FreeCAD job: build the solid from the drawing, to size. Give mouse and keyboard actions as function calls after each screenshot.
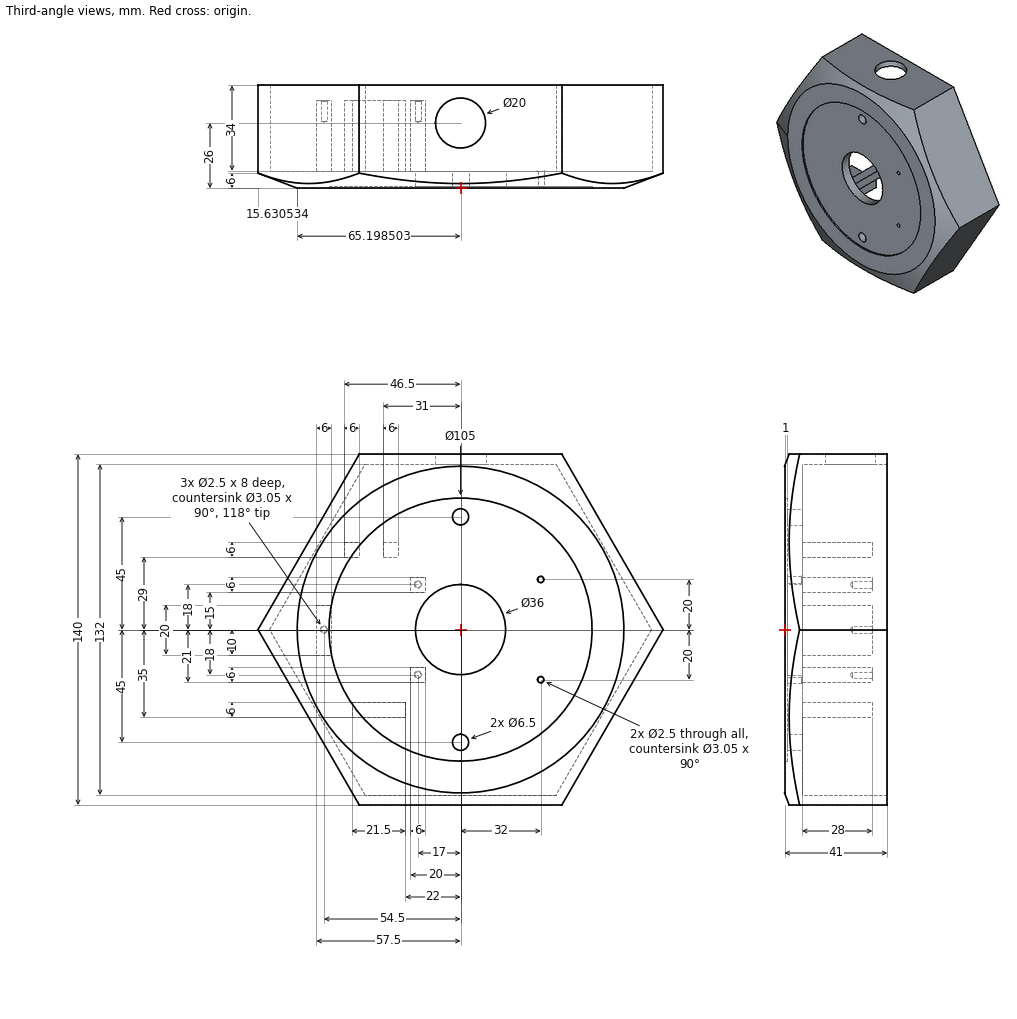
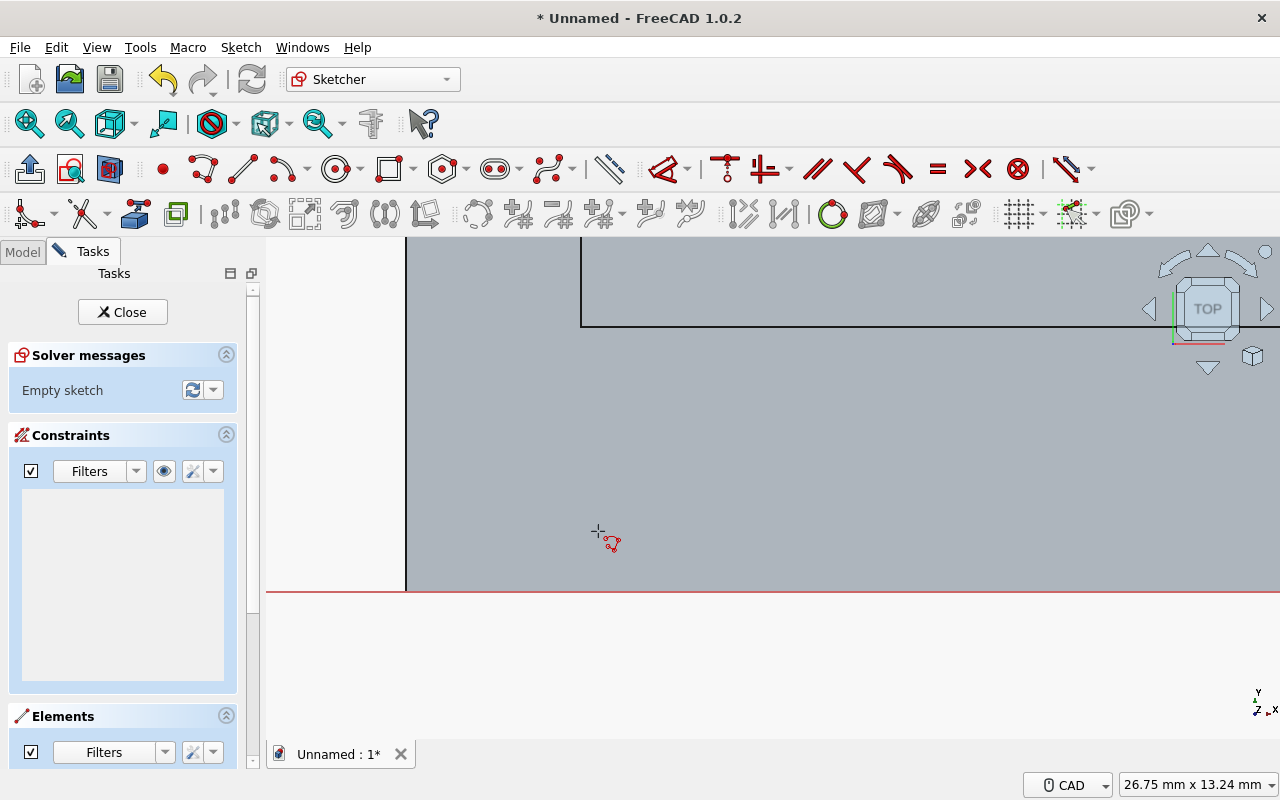
click(999, 592)
click(406, 365)
click(406, 583)
click(999, 592)
key(Escape)
key(Escape)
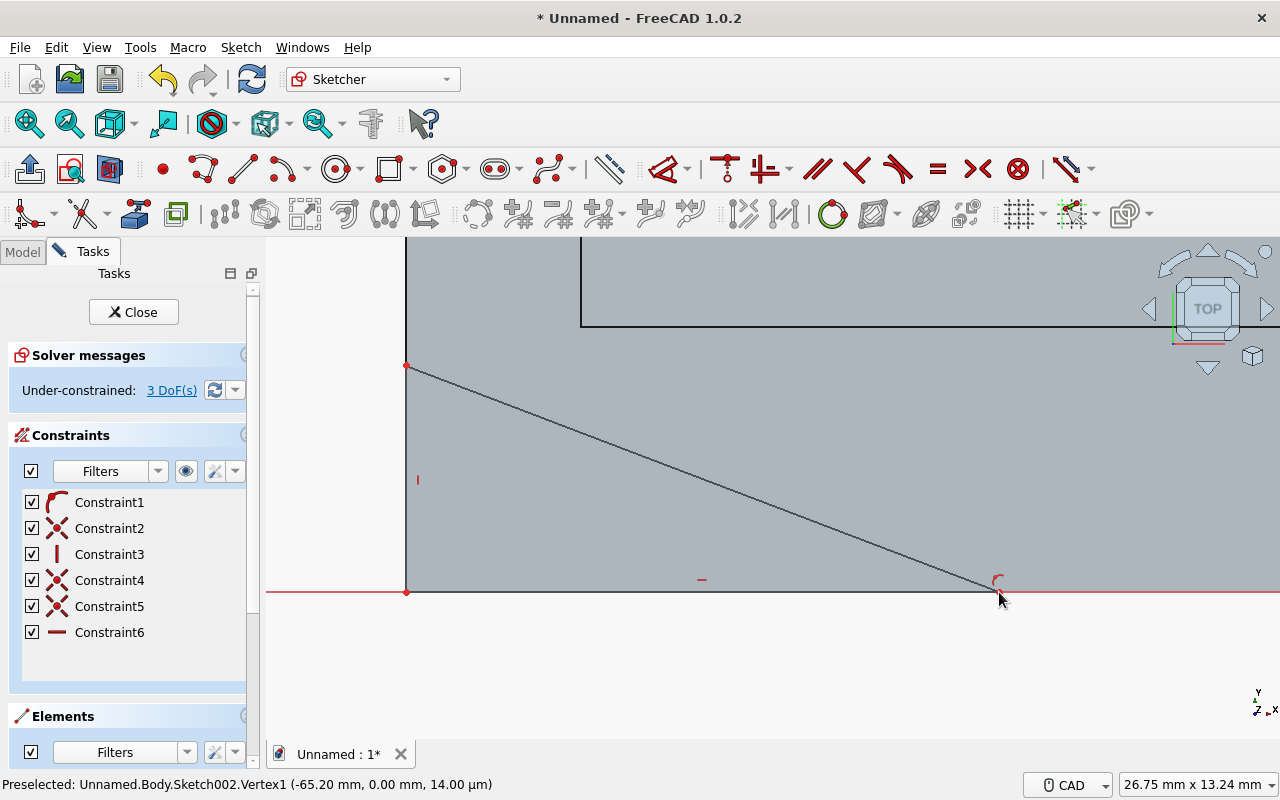
click(406, 434)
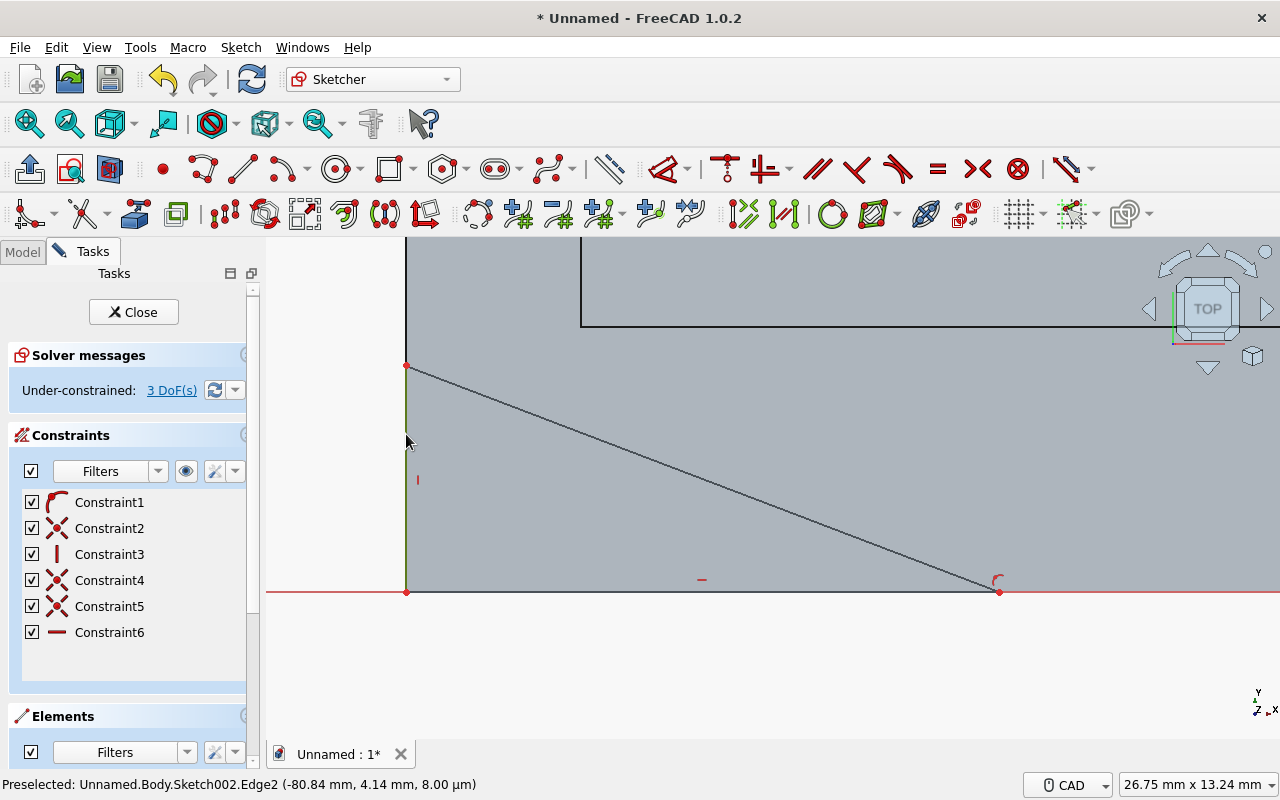
key(i)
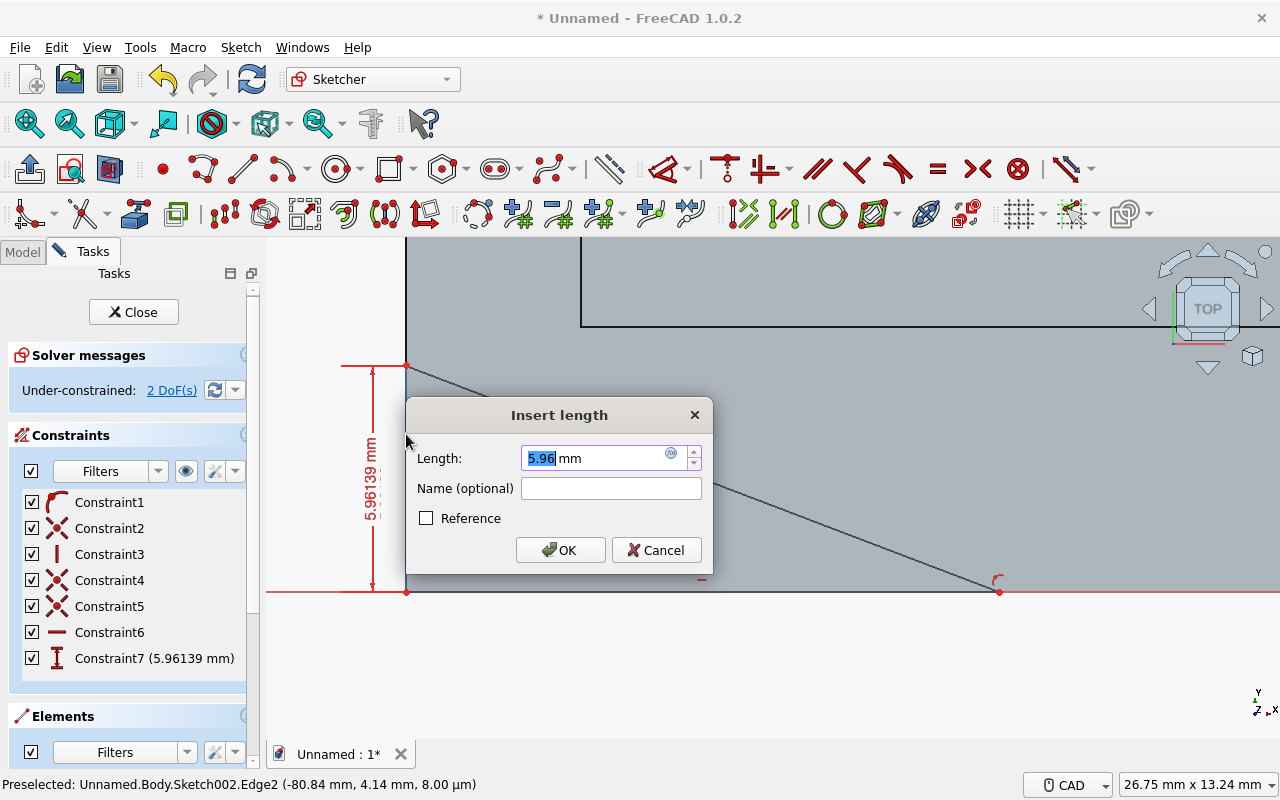
text(6)
key(Return)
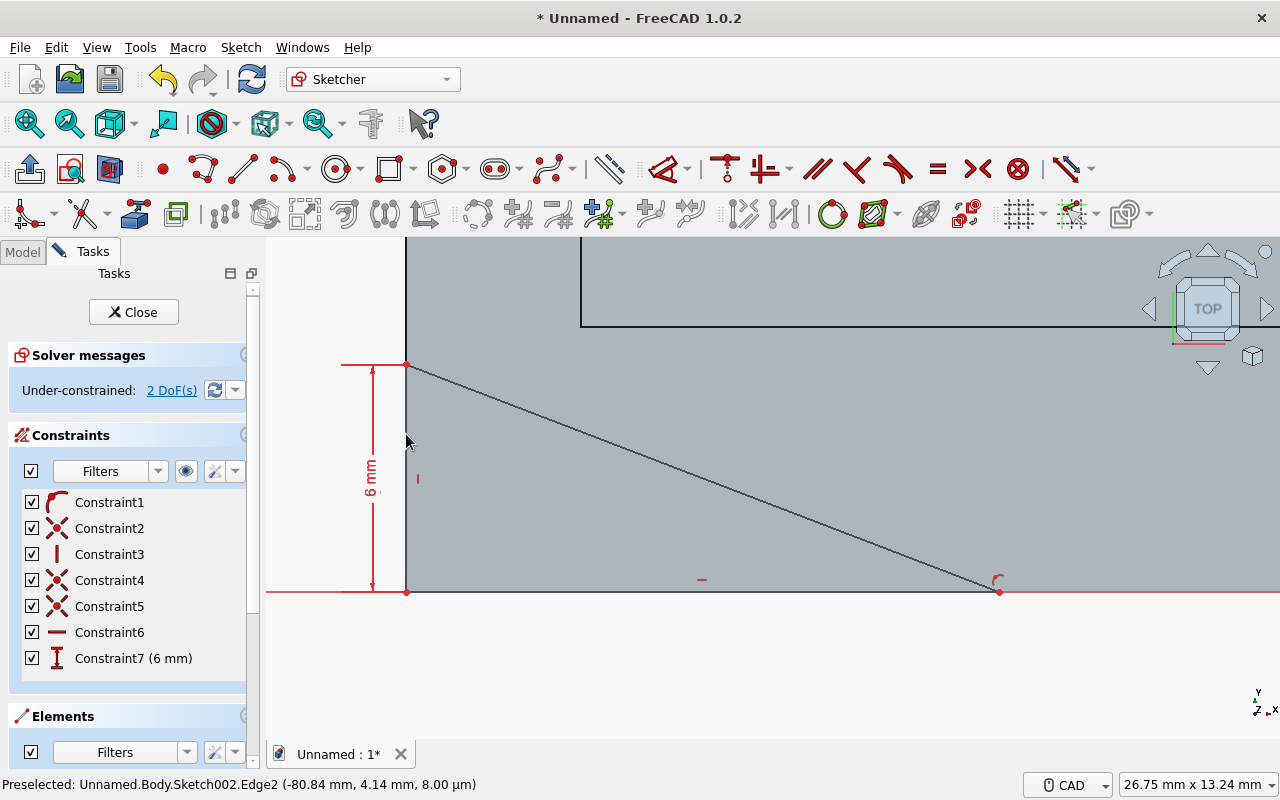
click(584, 592)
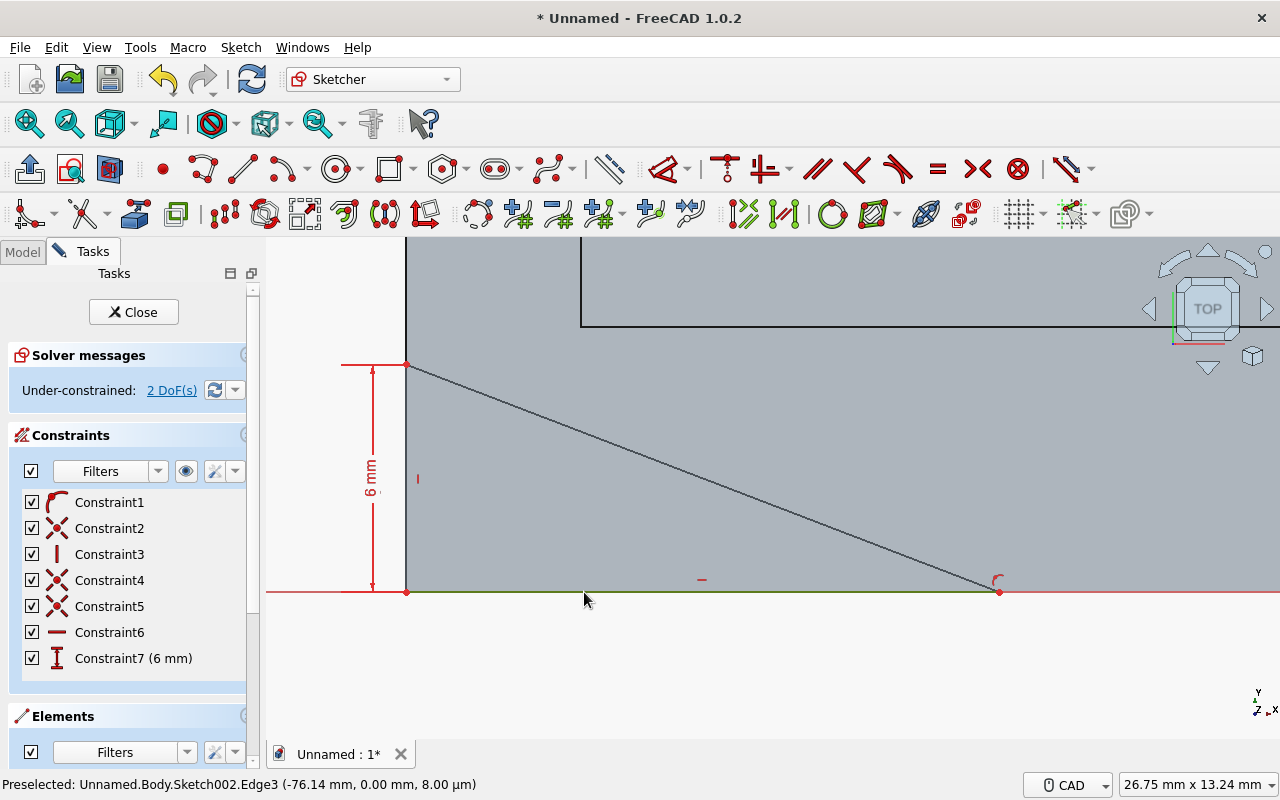
key(l)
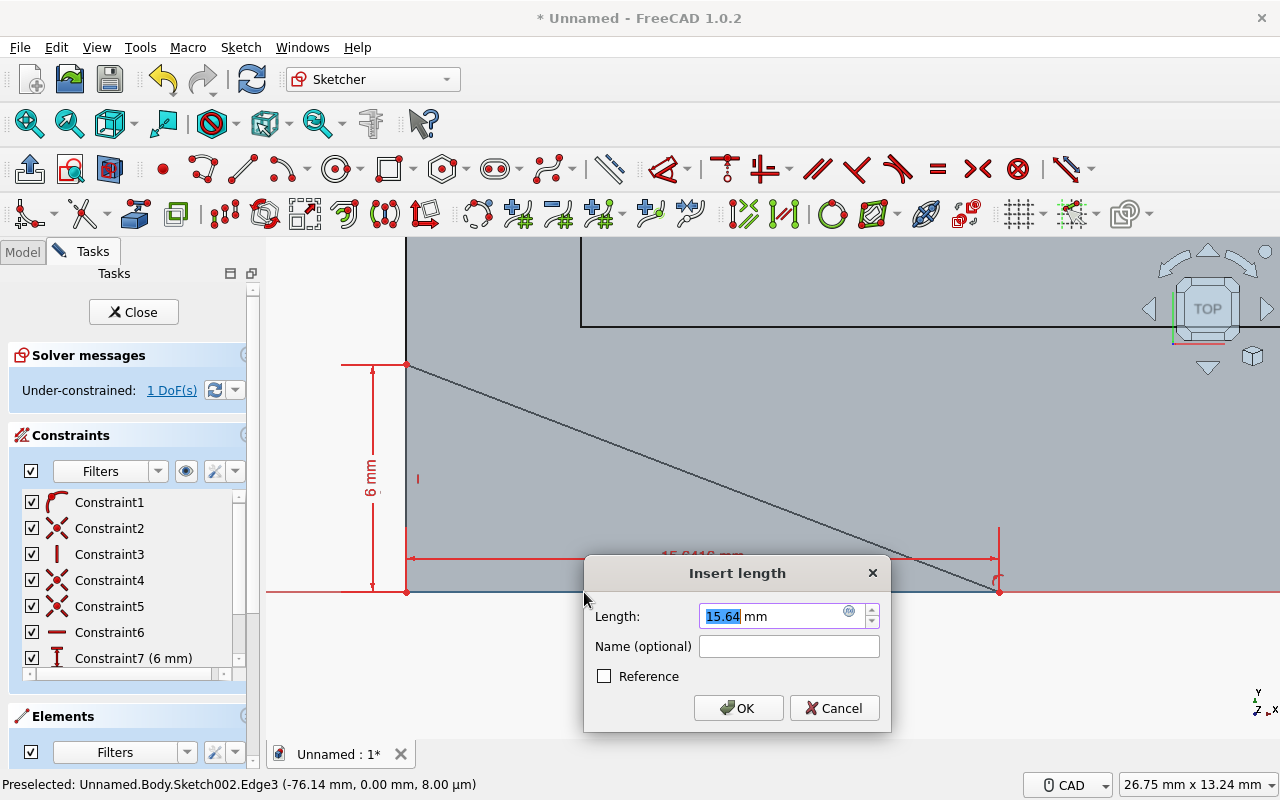
text(15.630534)
key(Return)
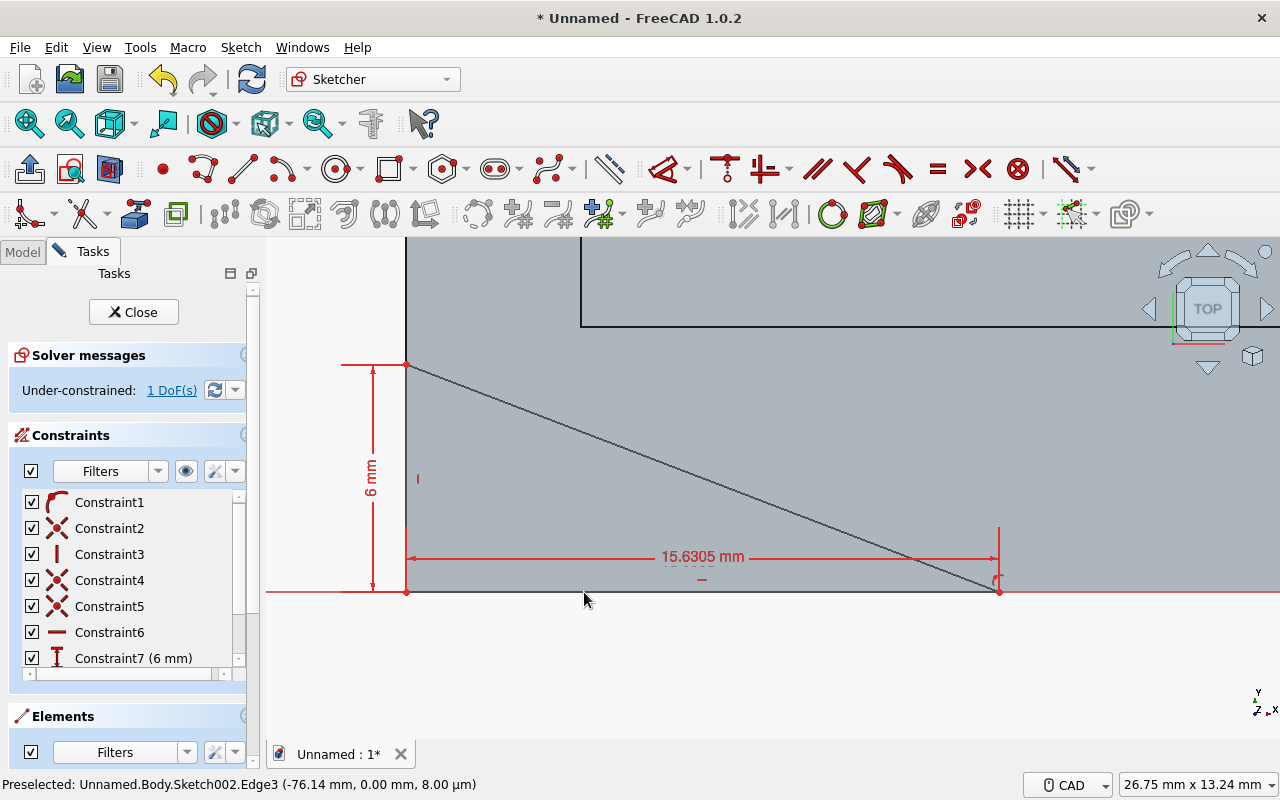
click(999, 592)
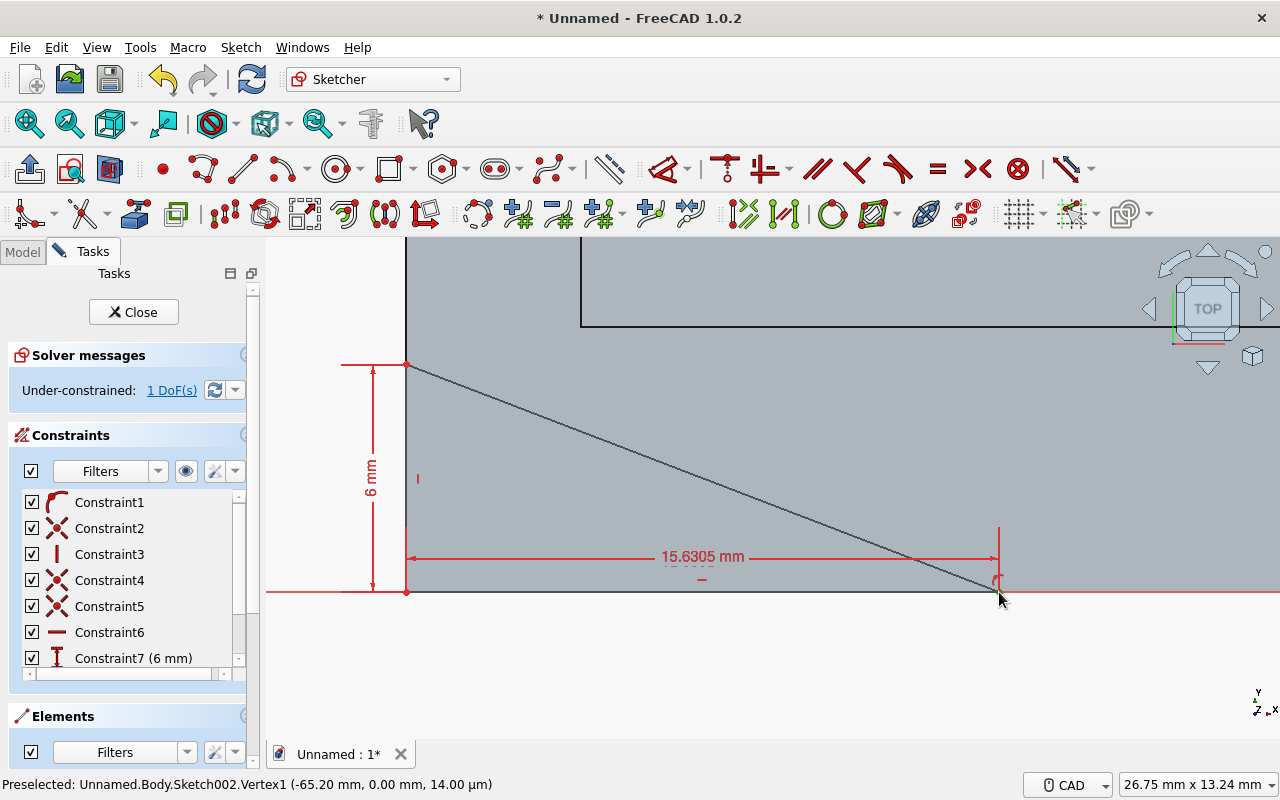
key(l)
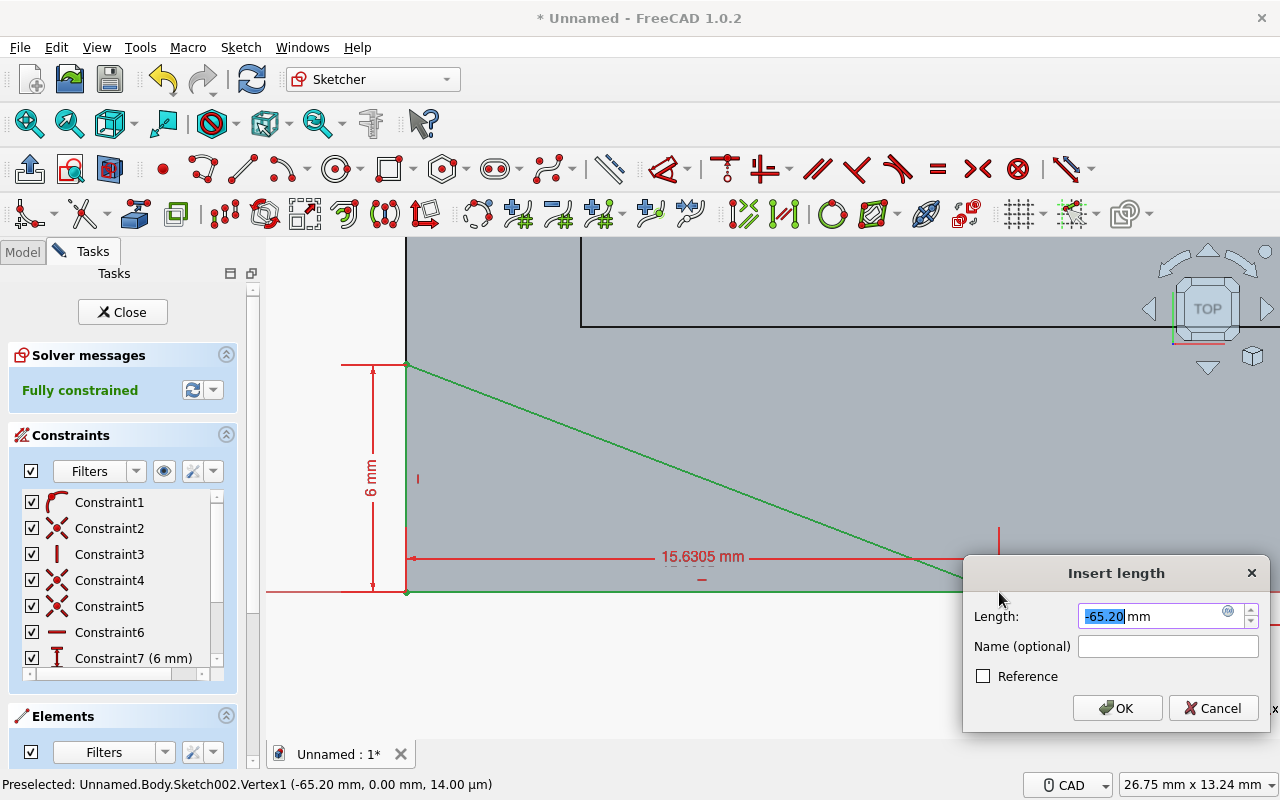
text(-65.198503)
key(Return)